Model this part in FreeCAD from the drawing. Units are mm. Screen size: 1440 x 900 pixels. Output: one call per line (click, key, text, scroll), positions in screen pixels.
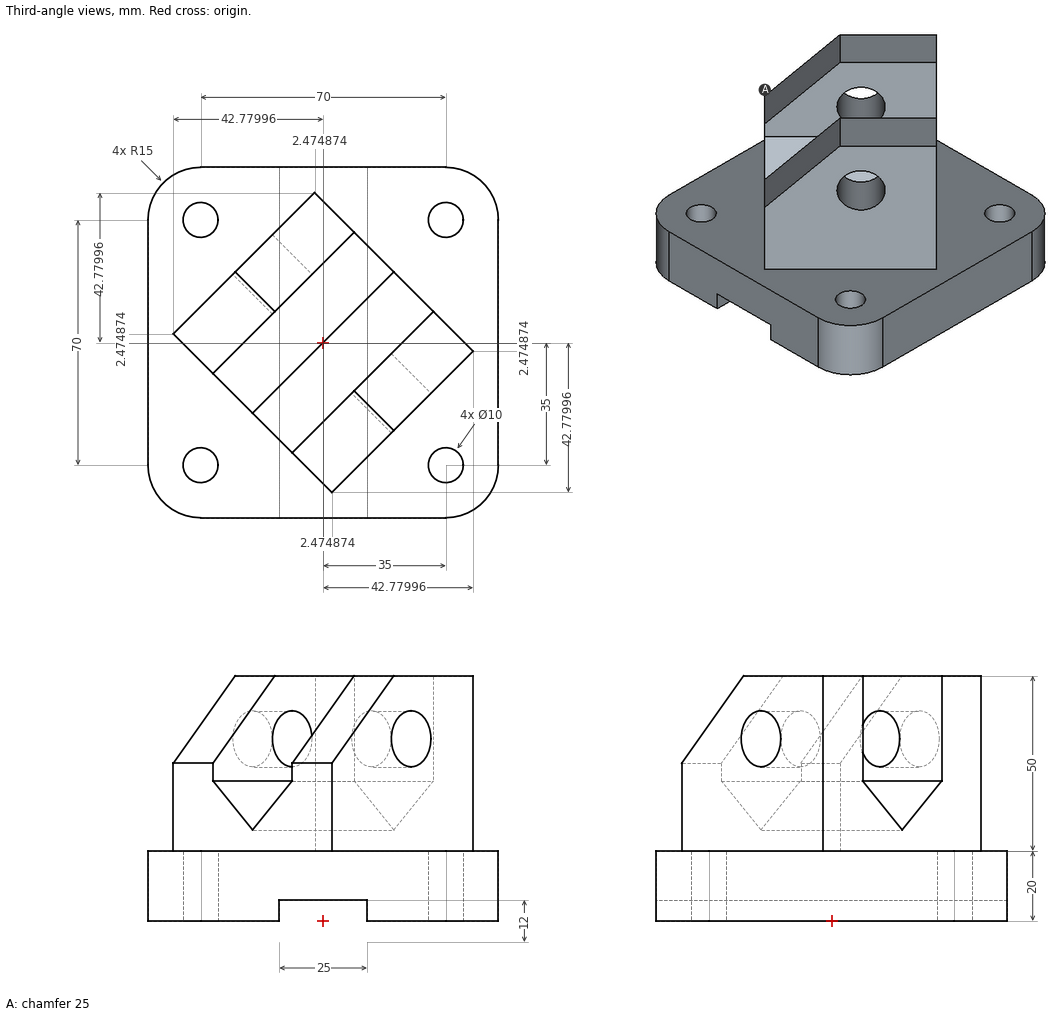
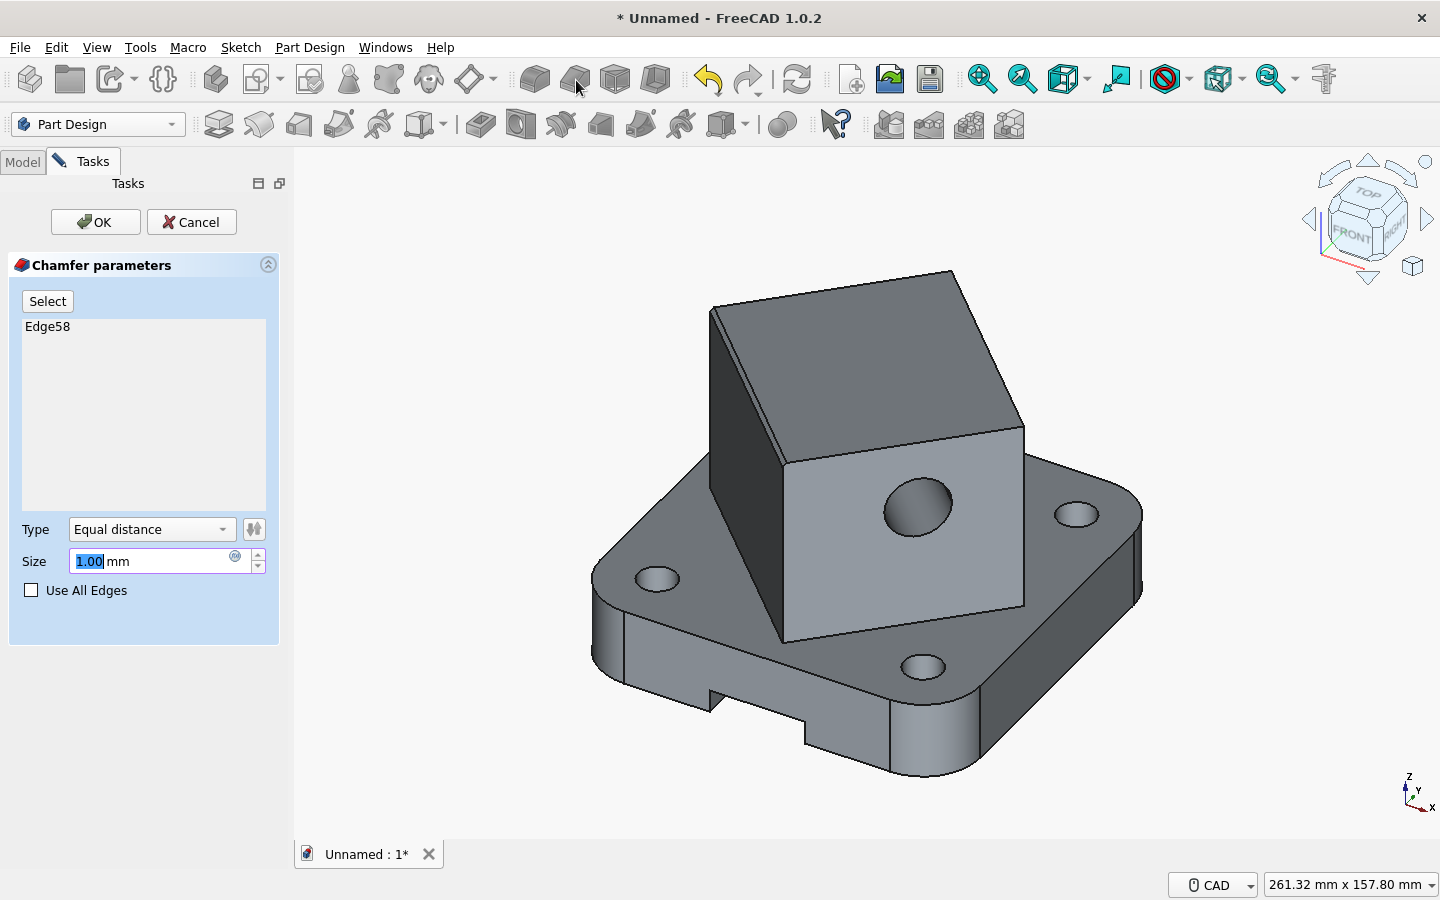
text(25)
key(Tab)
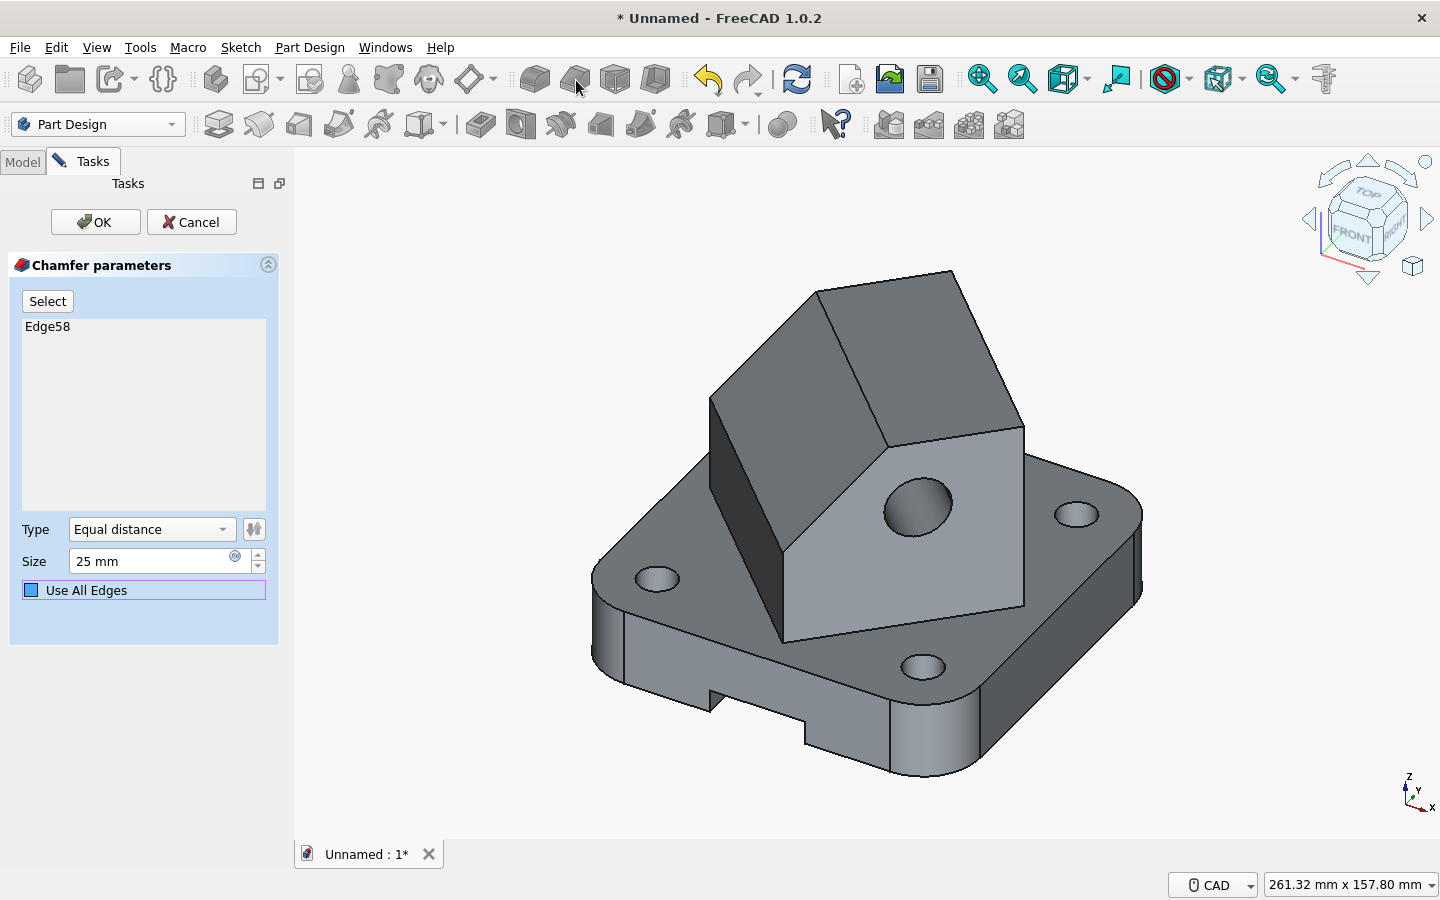
click(96, 222)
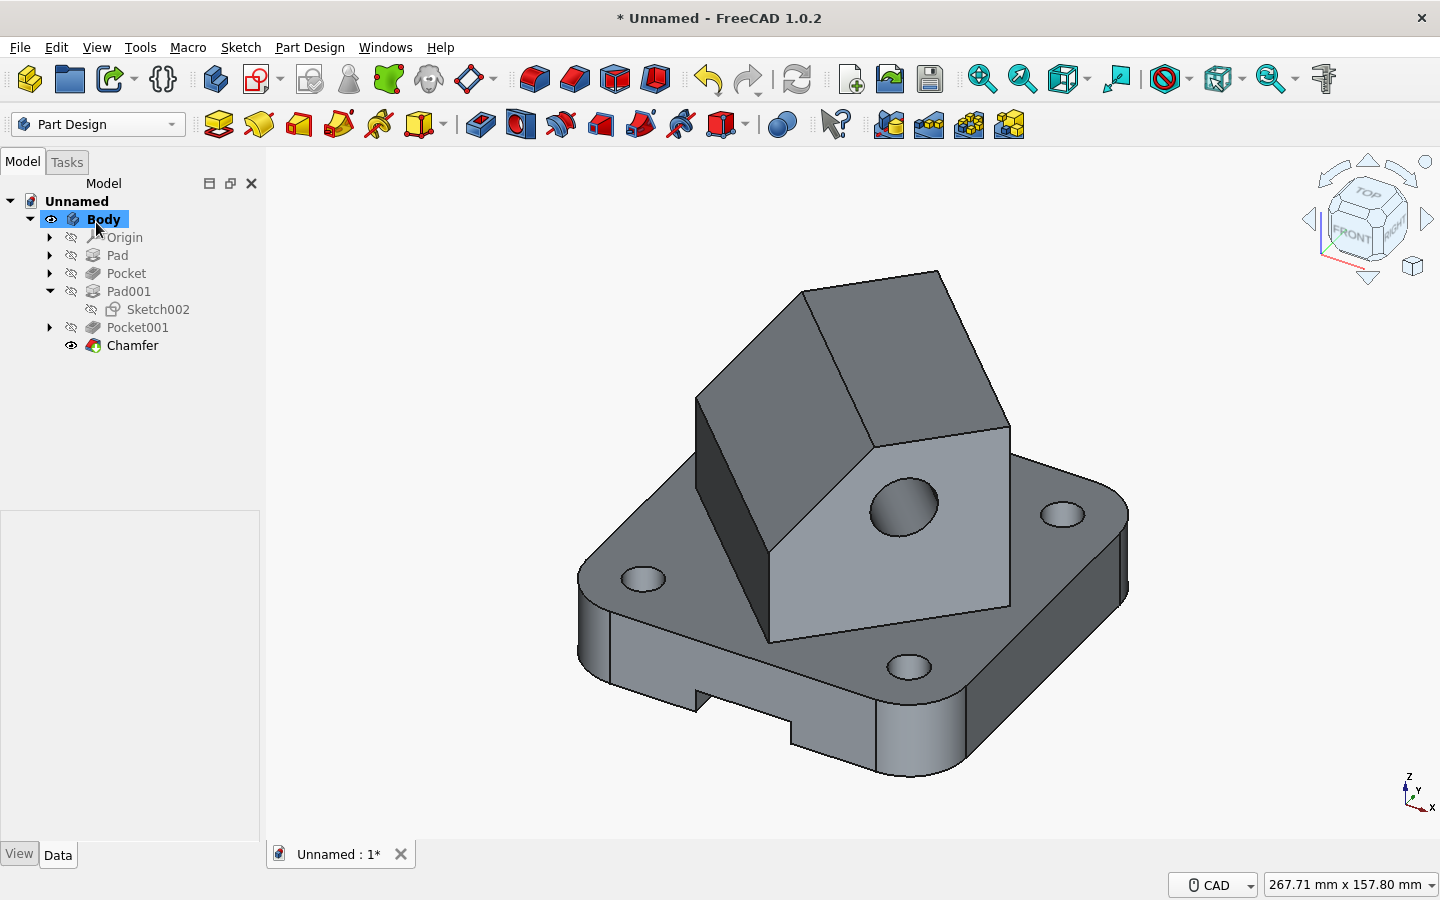
key(3)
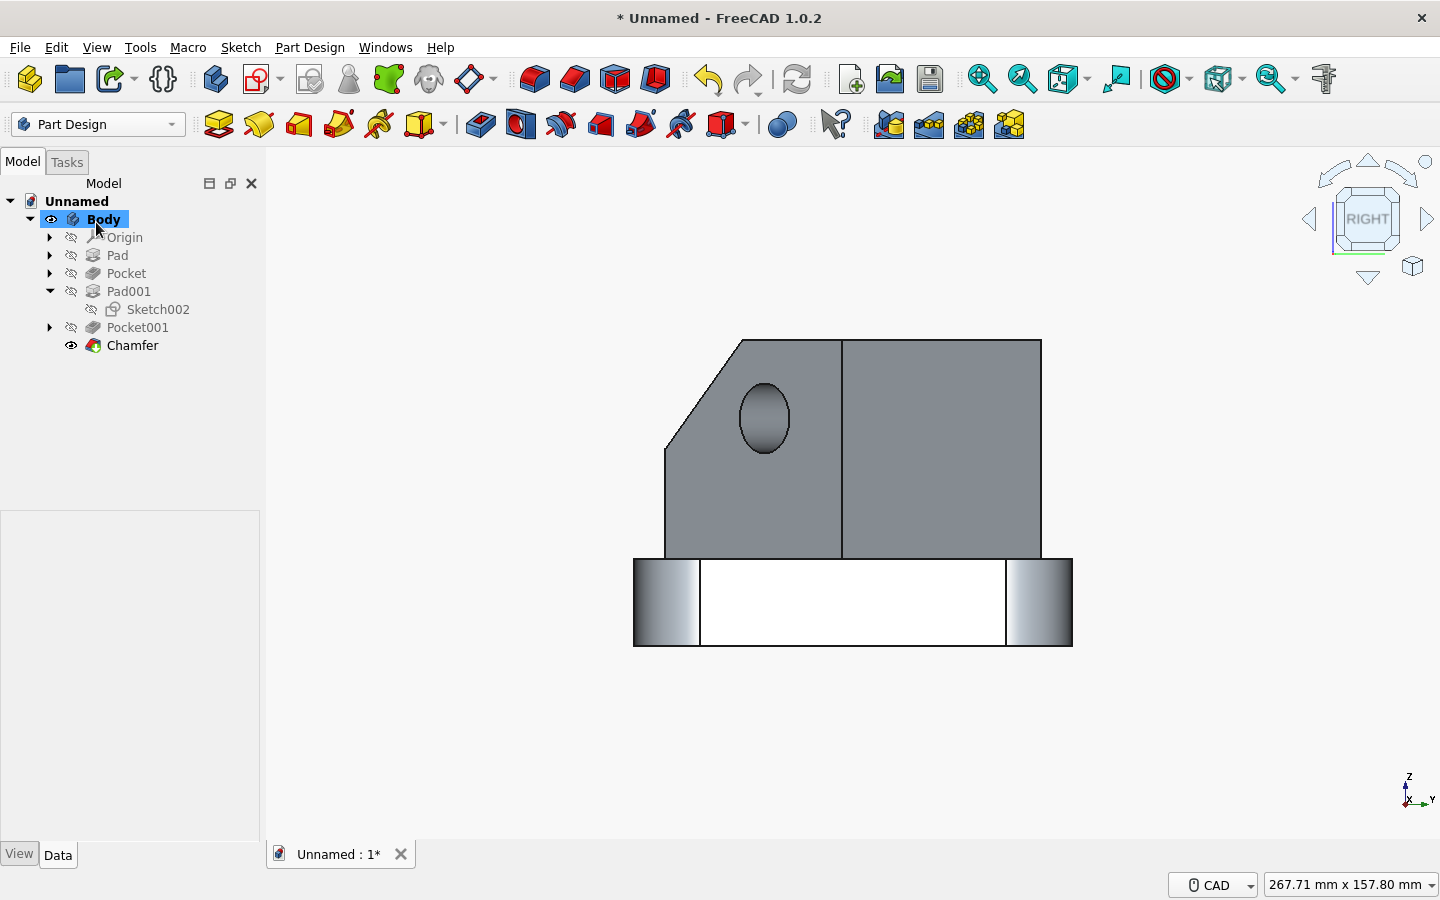
key(v)
key(f)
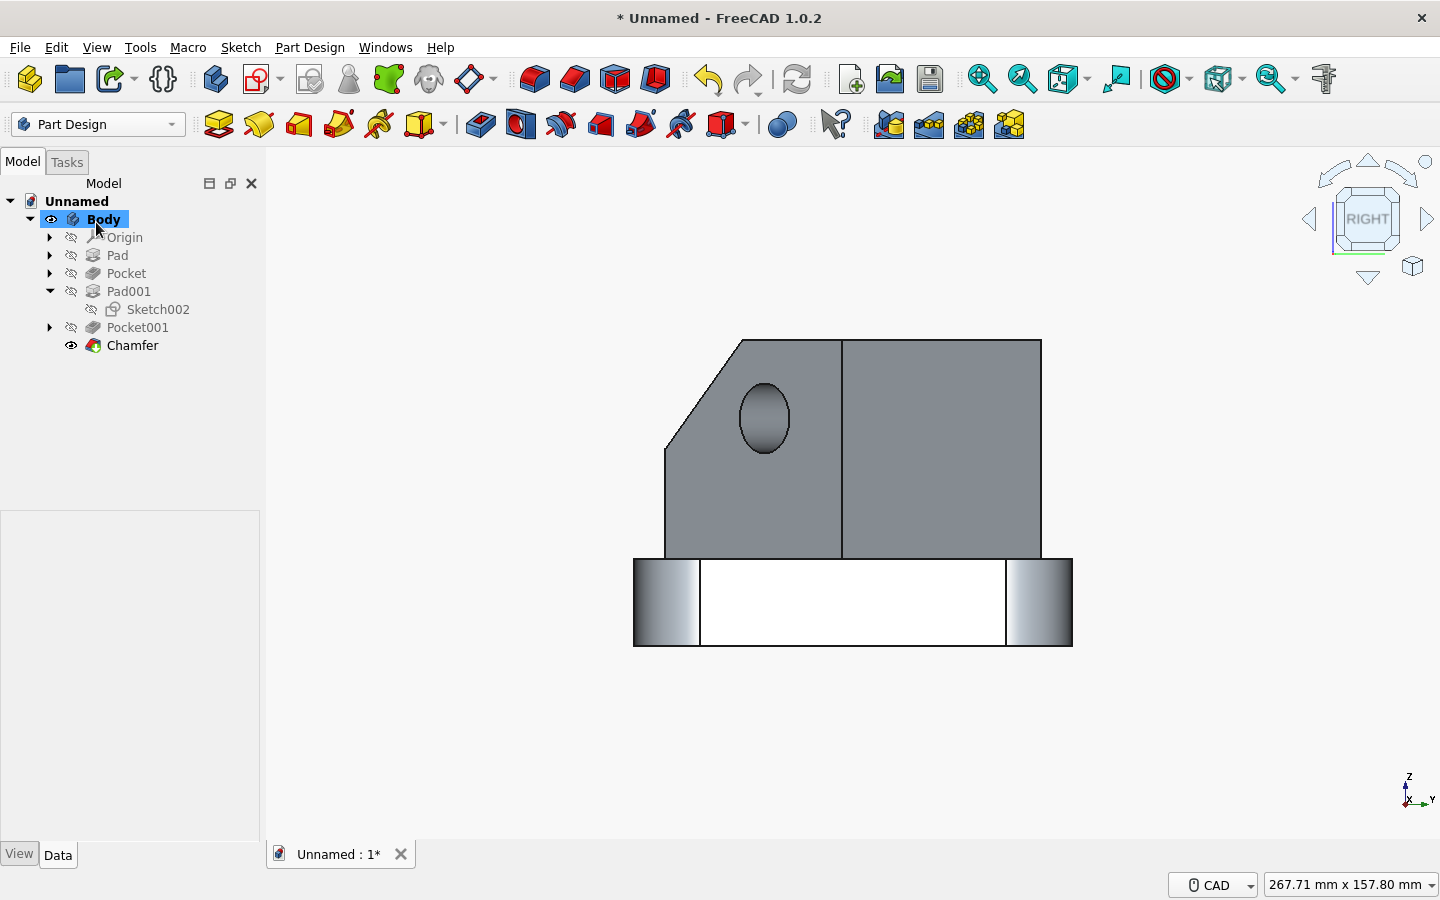
click(941, 448)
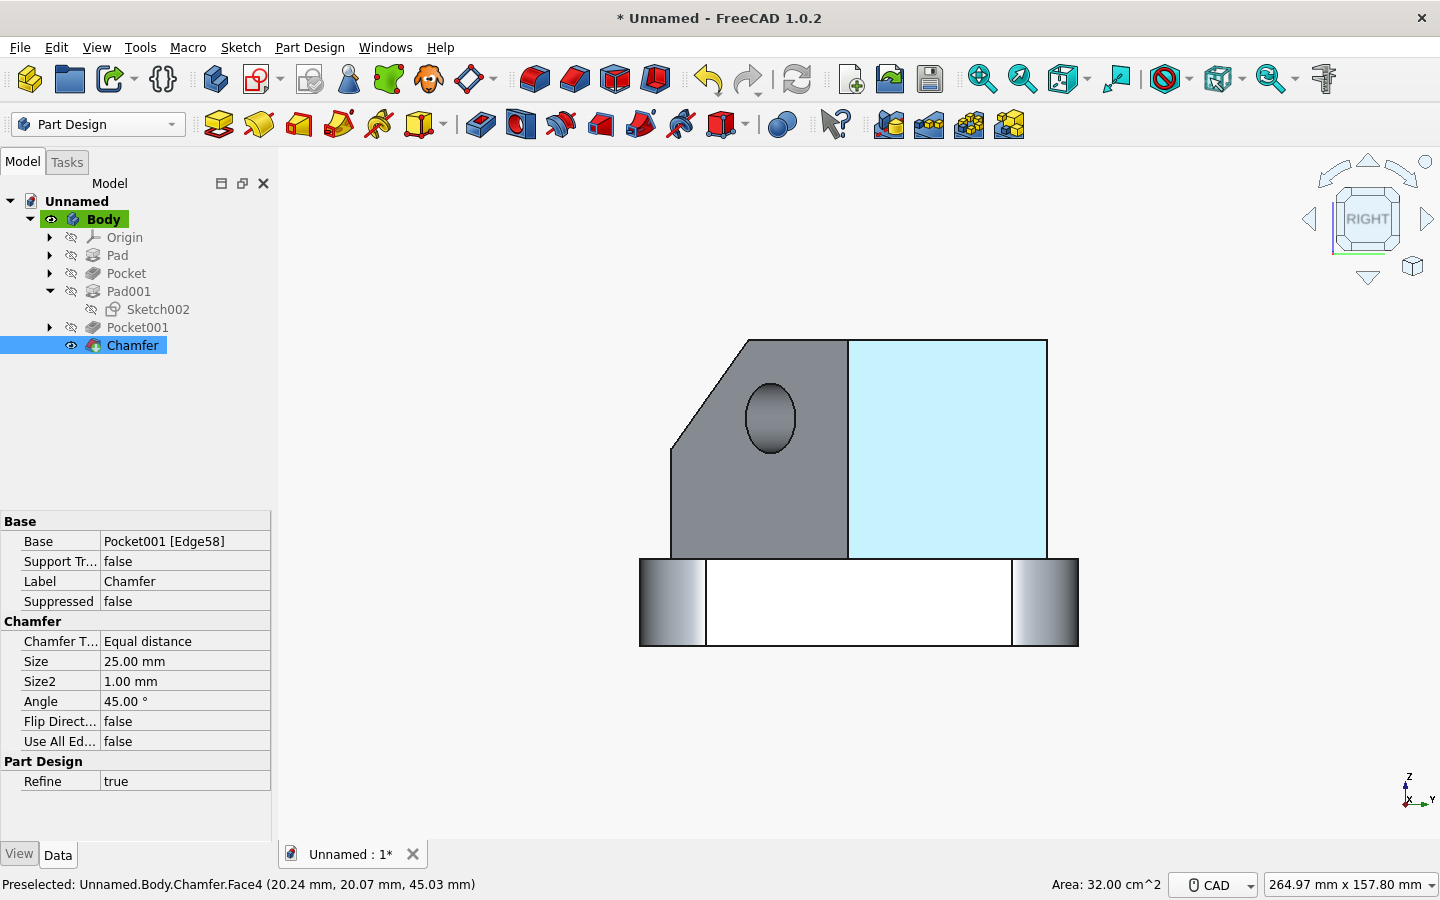
click(256, 80)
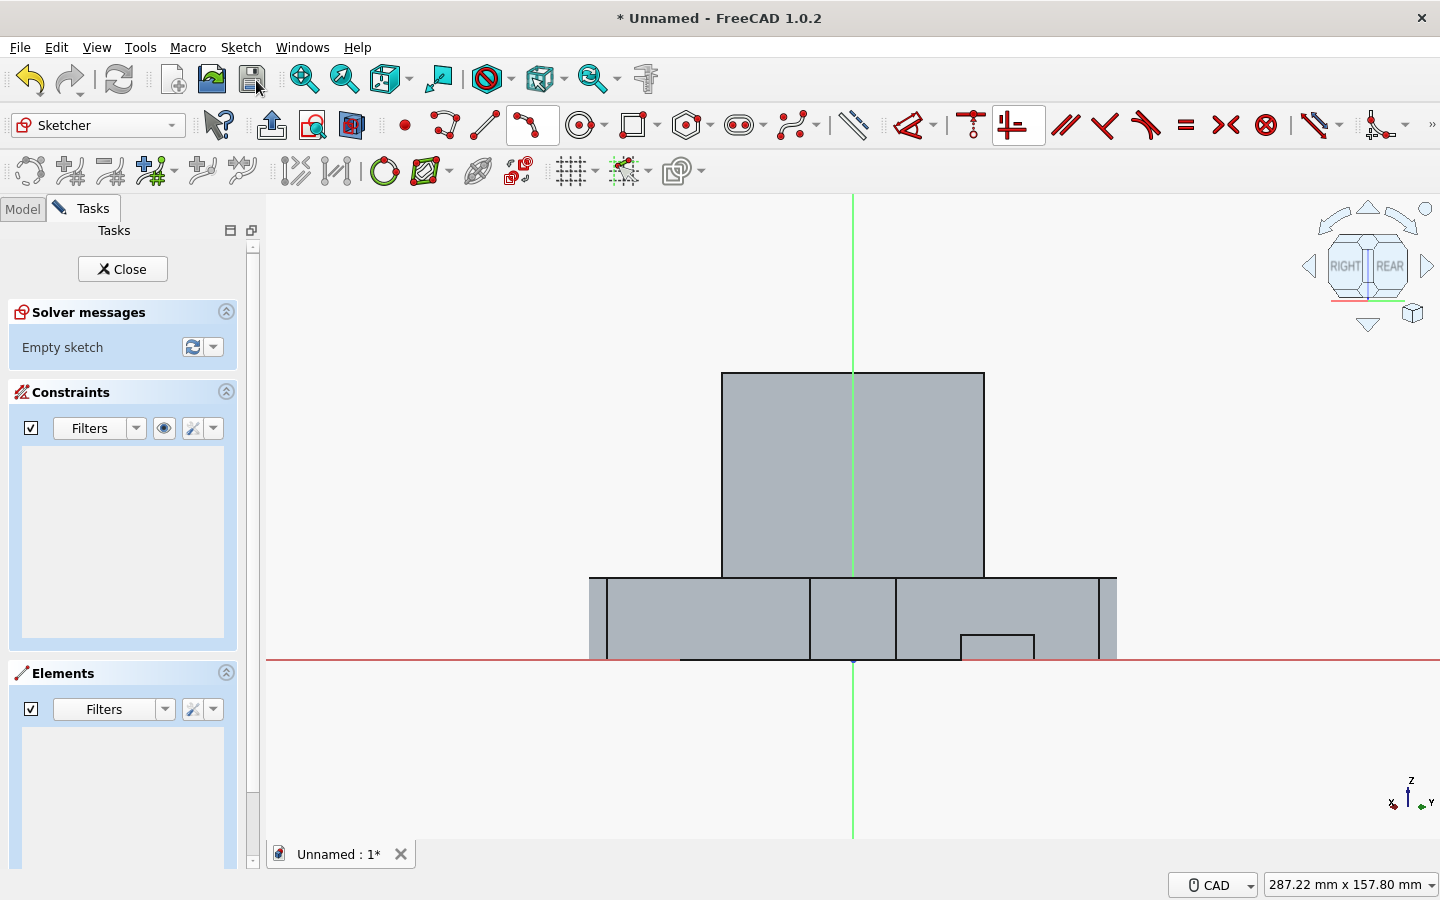
click(352, 126)